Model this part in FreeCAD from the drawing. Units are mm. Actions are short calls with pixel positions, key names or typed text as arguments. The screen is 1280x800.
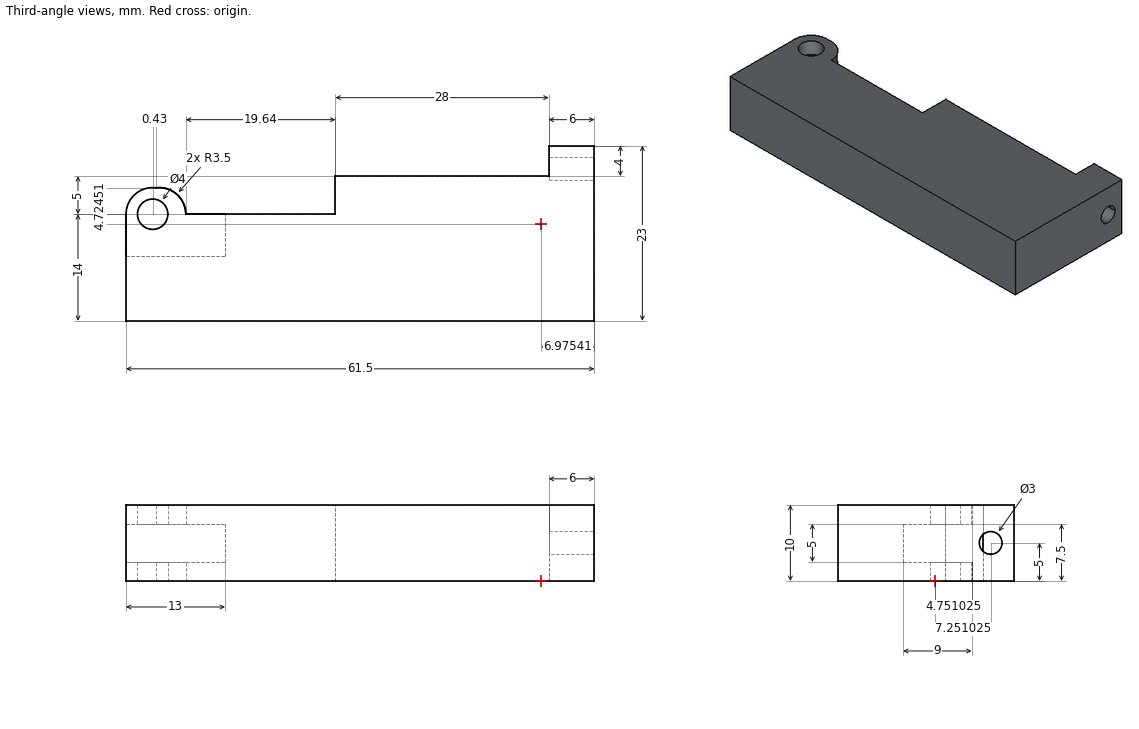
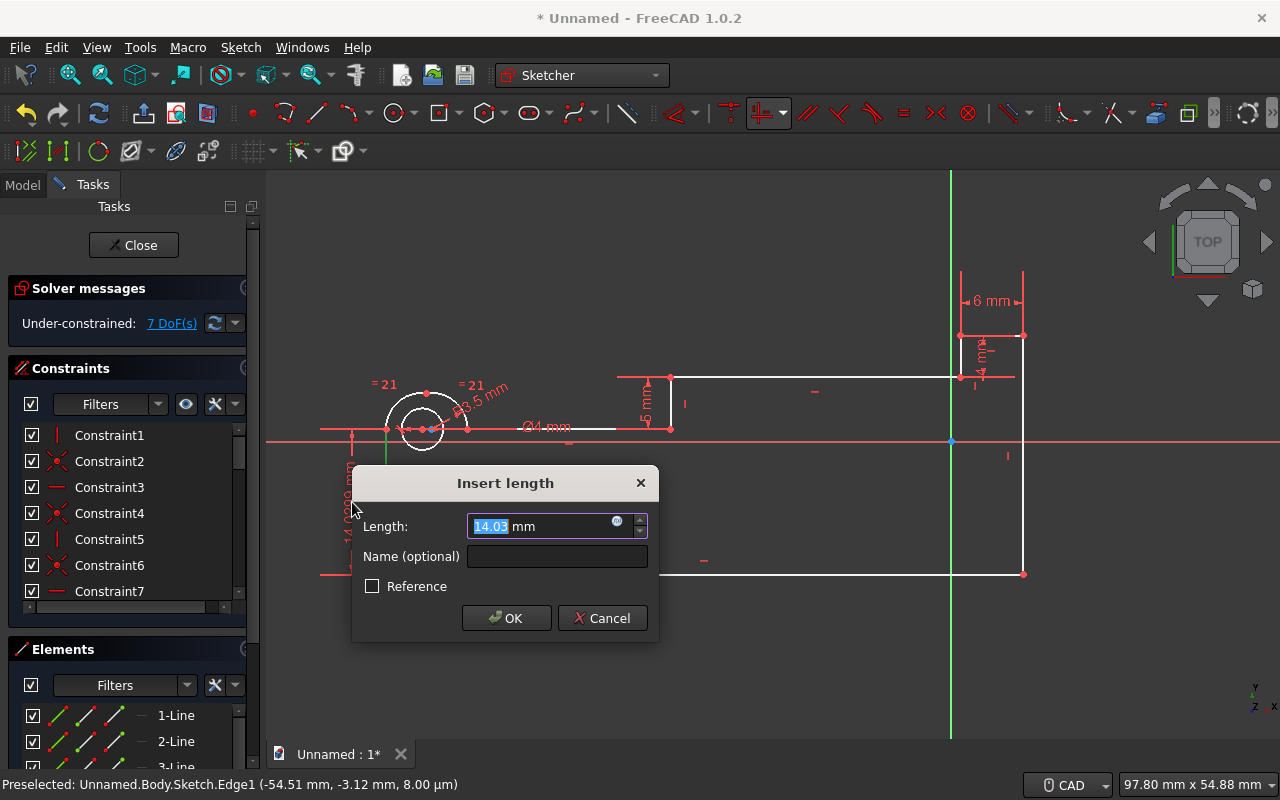
text(14)
key(Return)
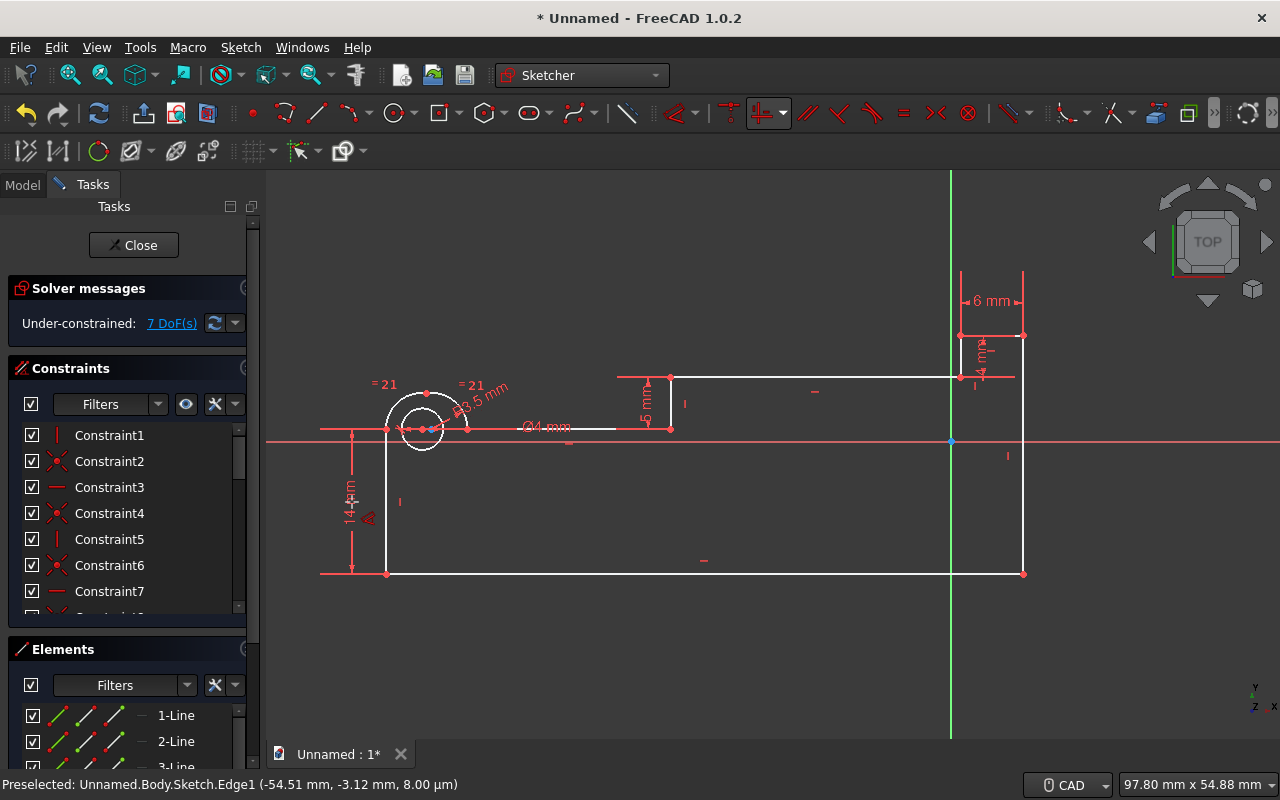
click(1023, 503)
click(1057, 455)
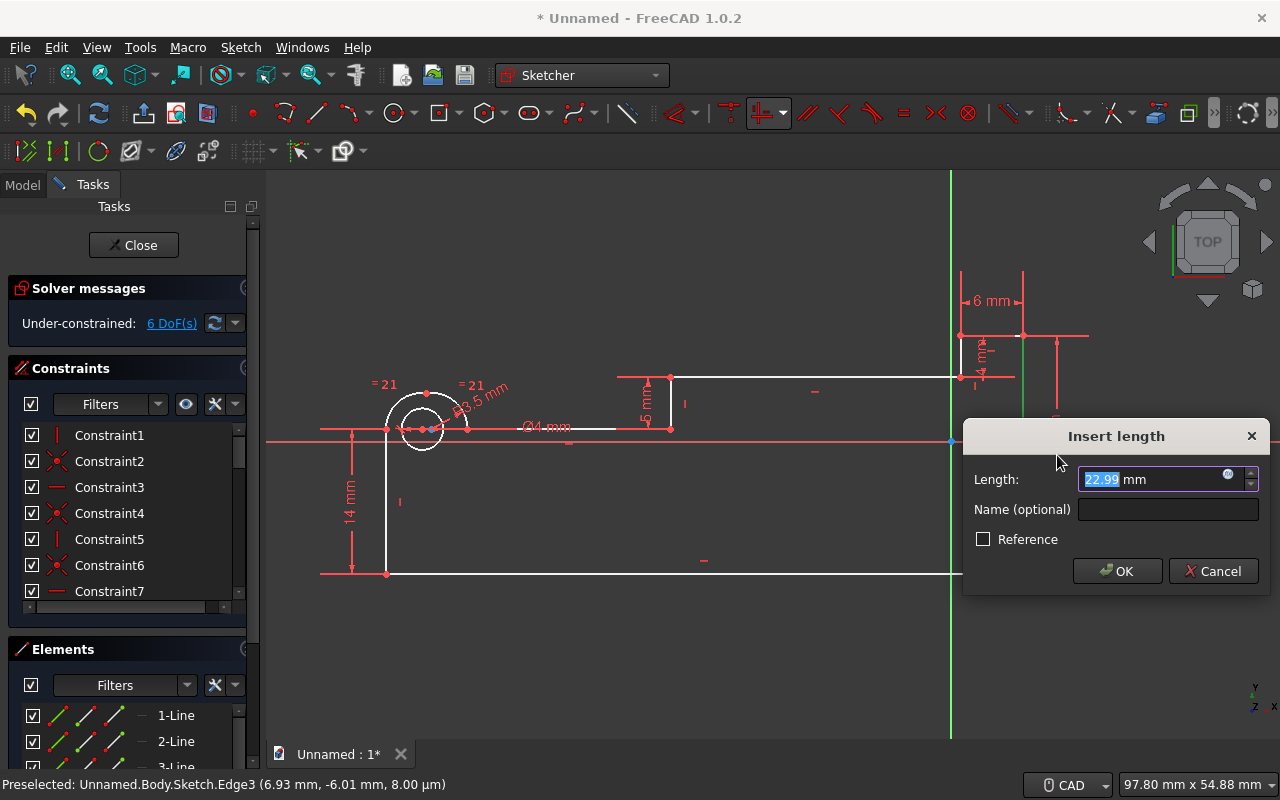
text(23)
key(Return)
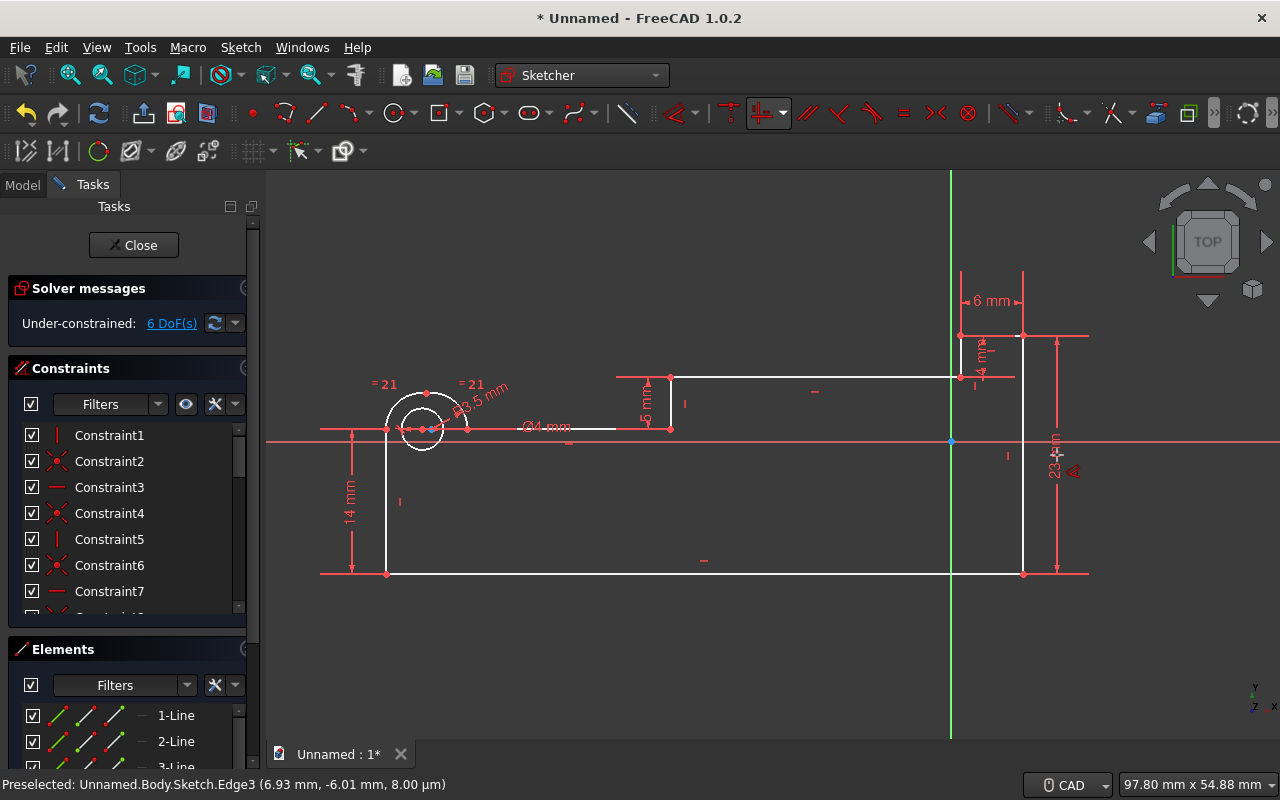
click(874, 377)
click(816, 343)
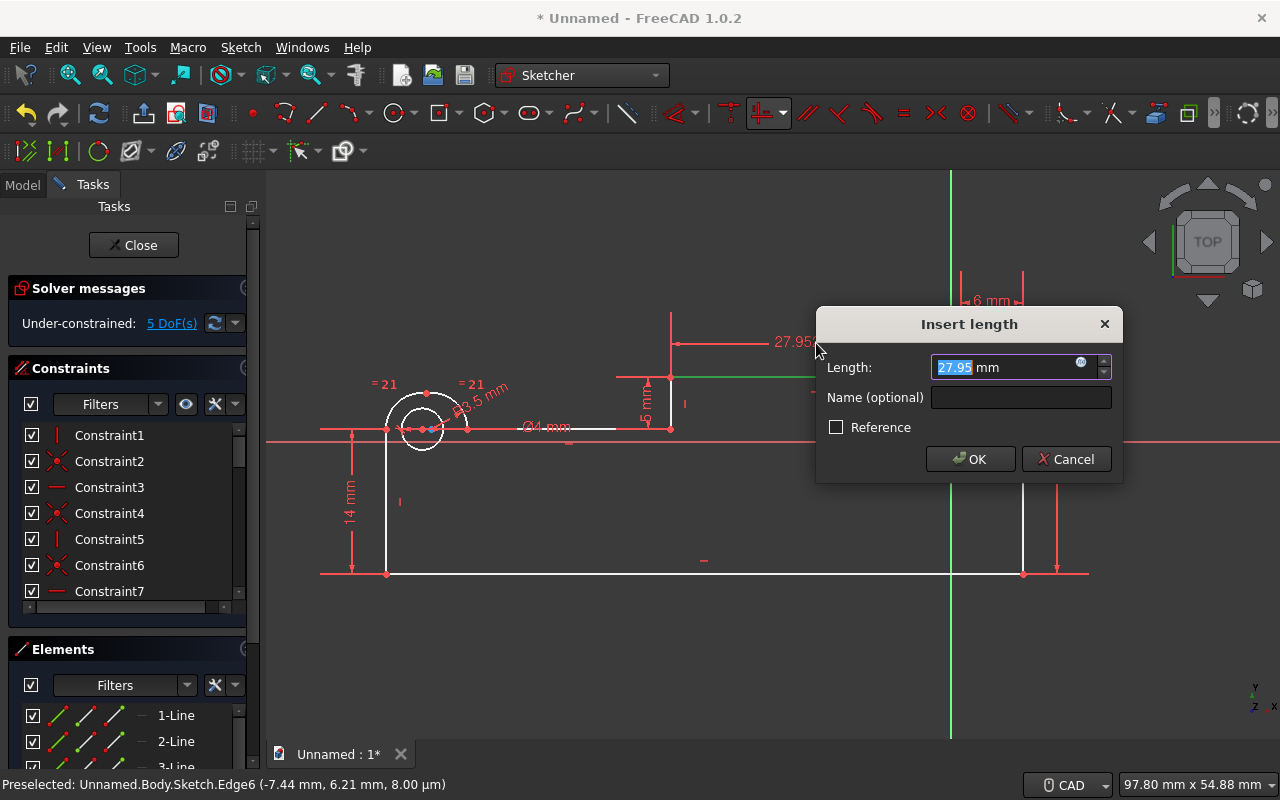
text(28)
key(Return)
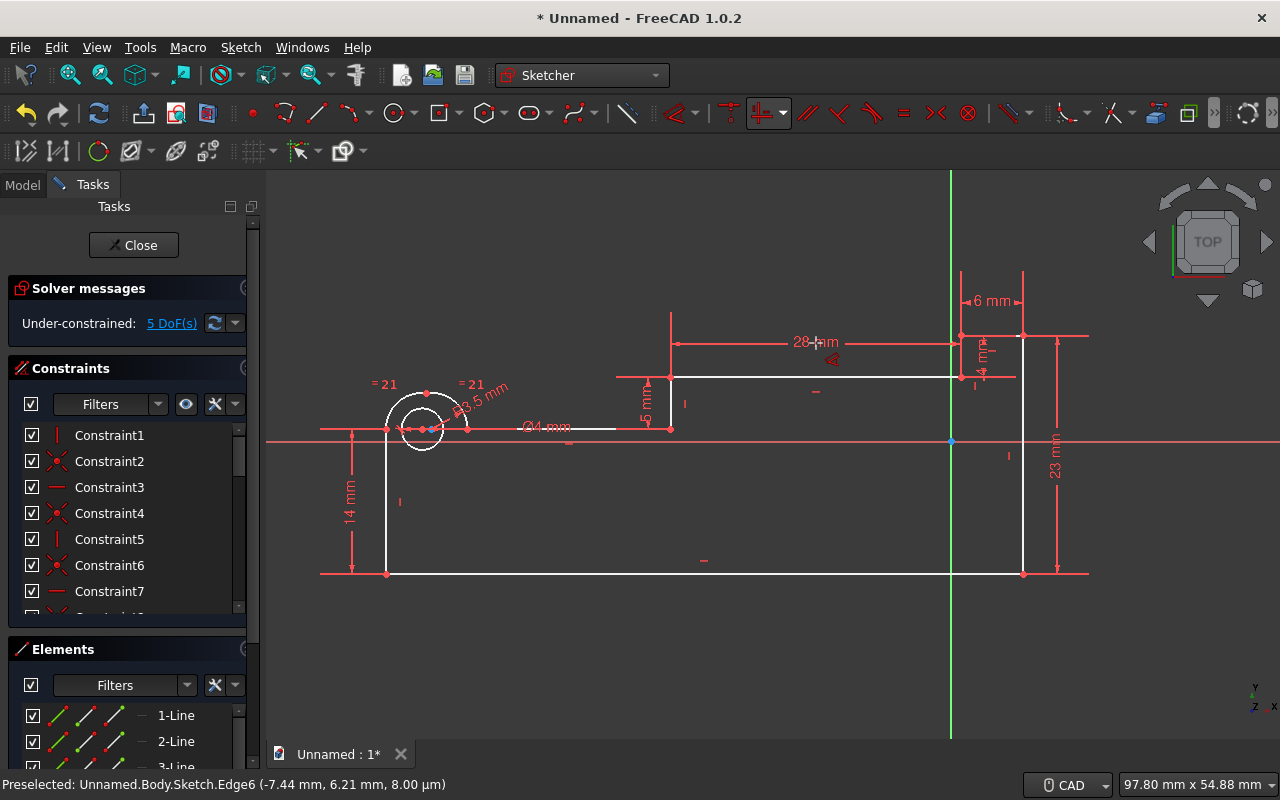
click(577, 574)
click(705, 608)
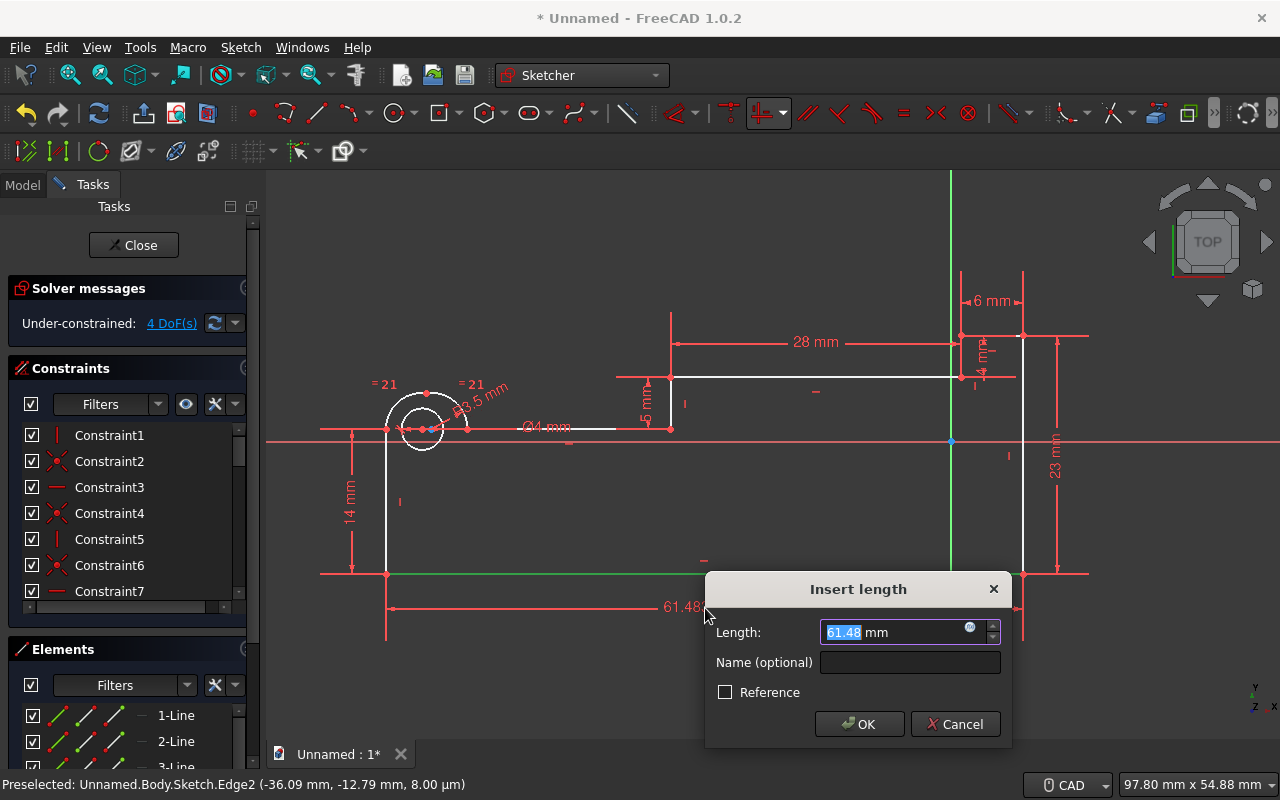
text(61.5)
key(Return)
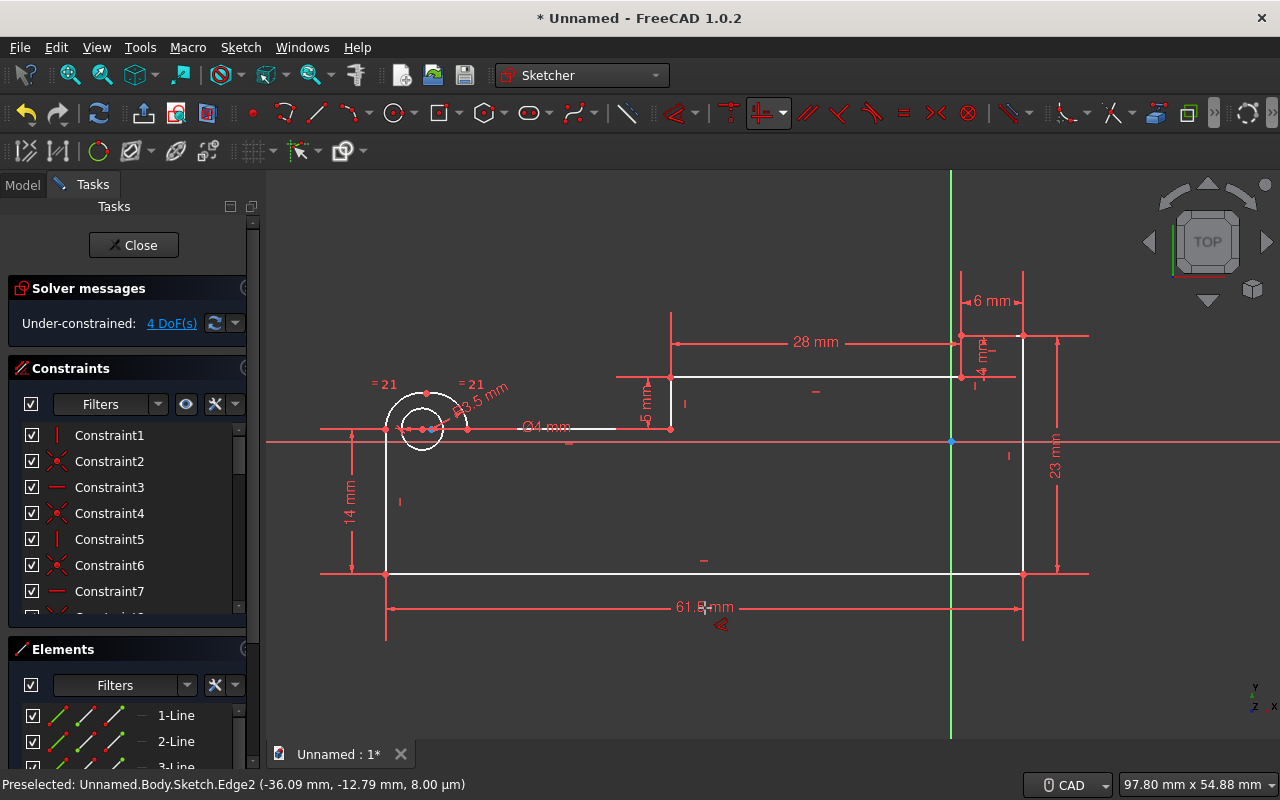
click(610, 429)
click(569, 395)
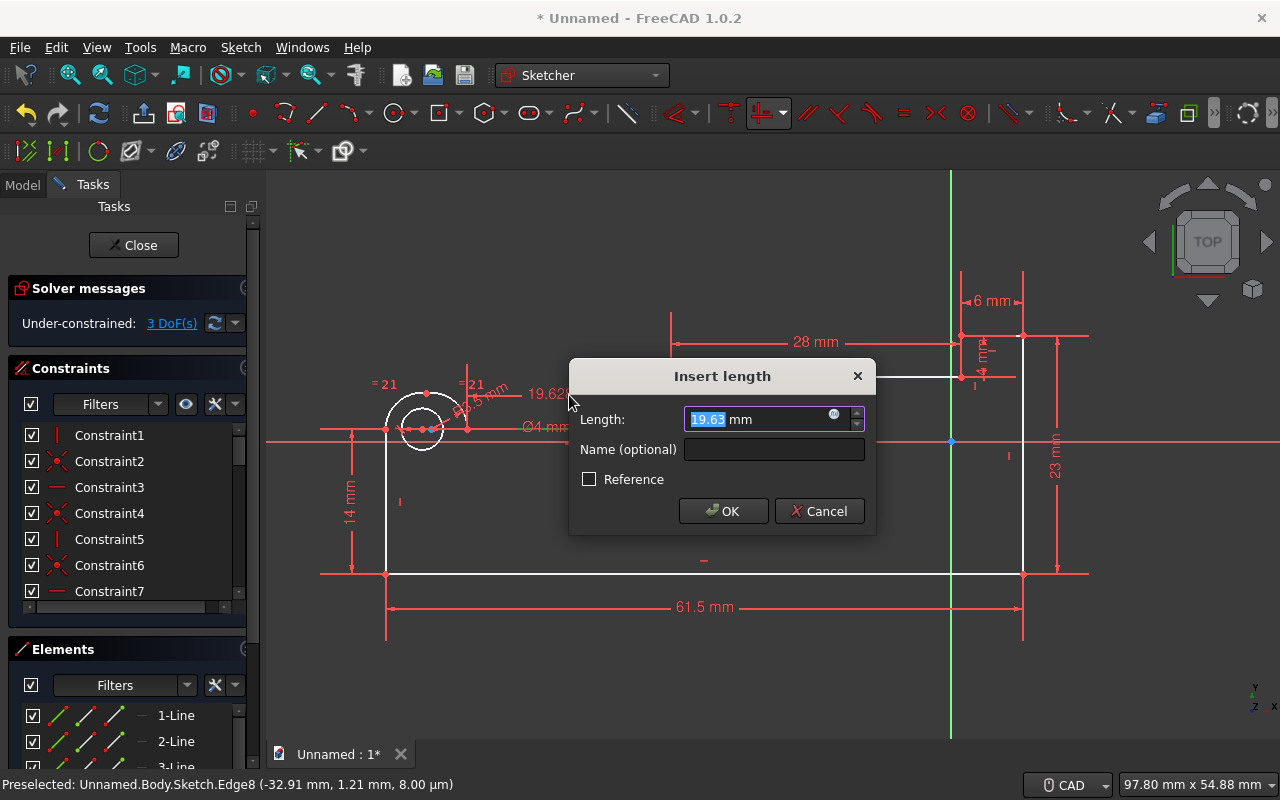
text(19.64)
key(Return)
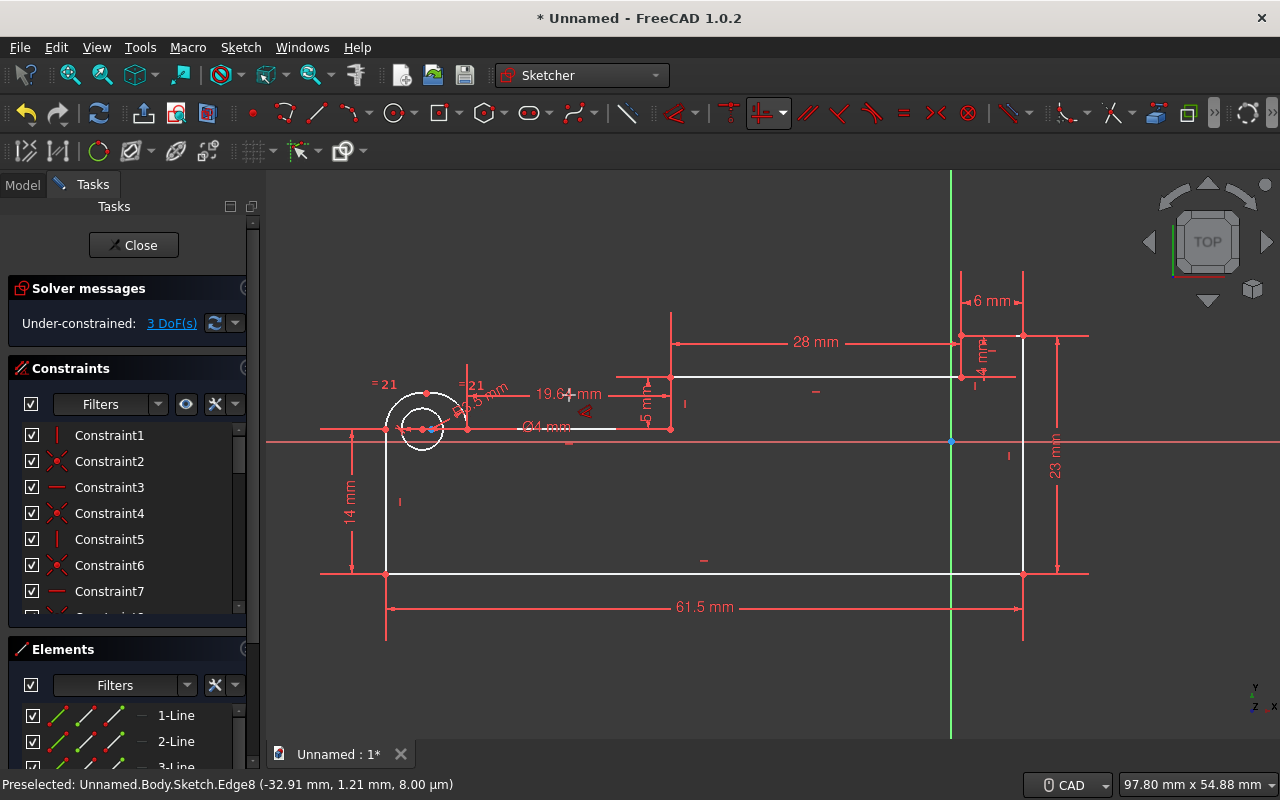
scroll(427, 393, up, 11)